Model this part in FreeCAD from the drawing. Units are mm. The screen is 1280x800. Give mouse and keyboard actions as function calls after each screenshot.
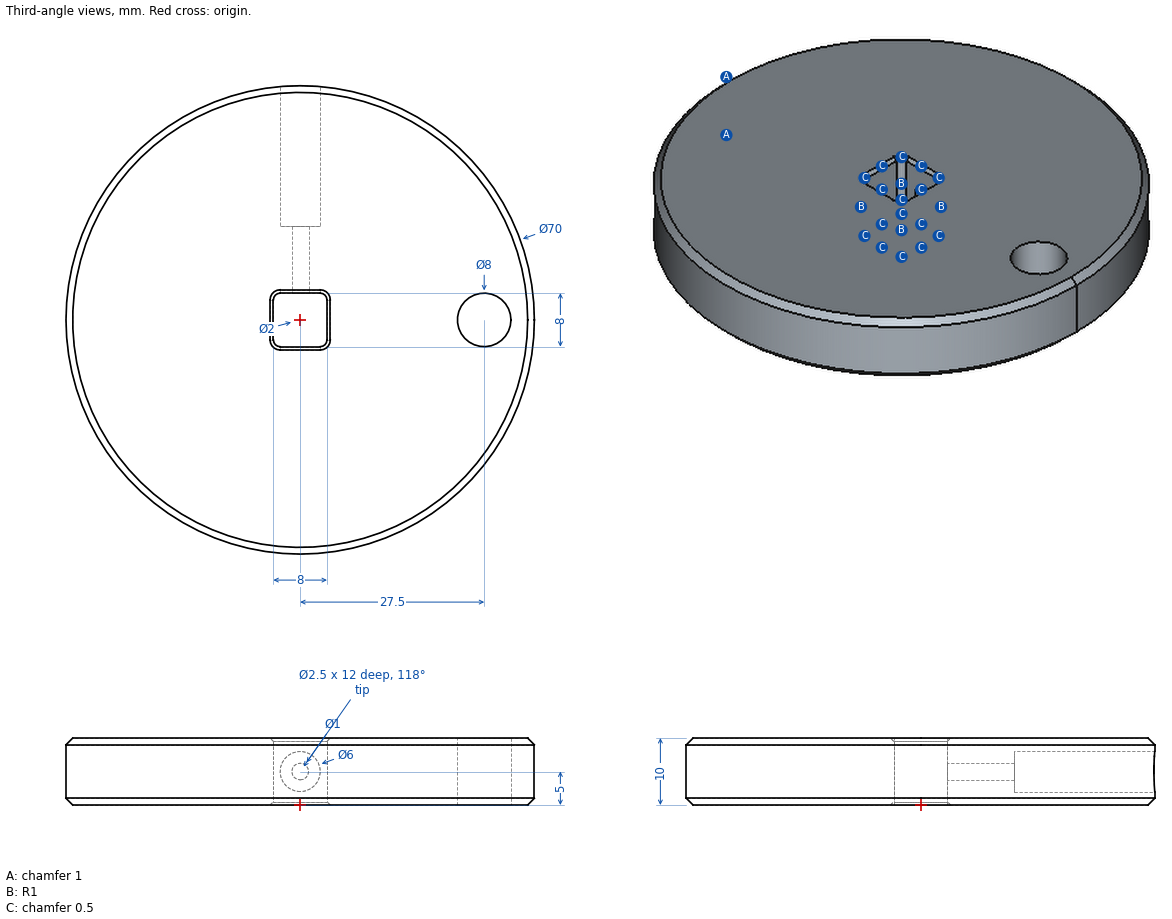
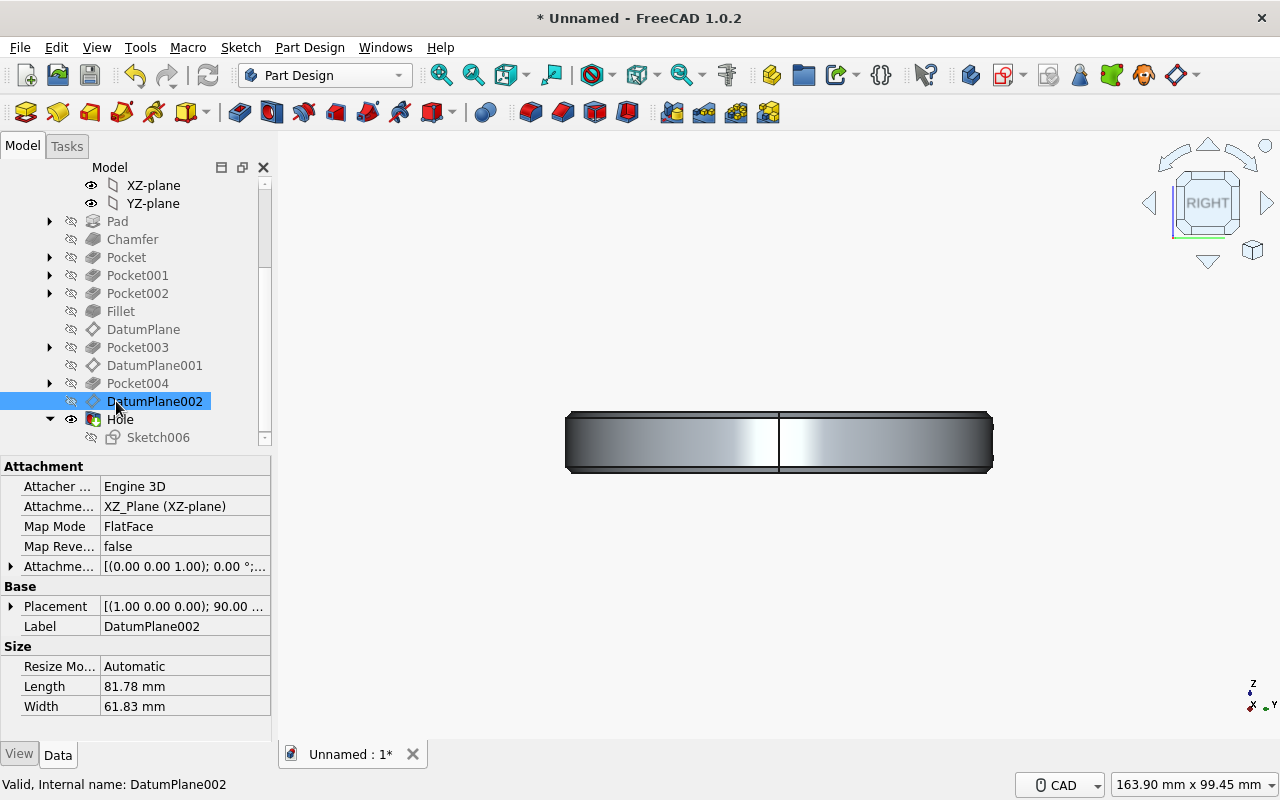
click(442, 76)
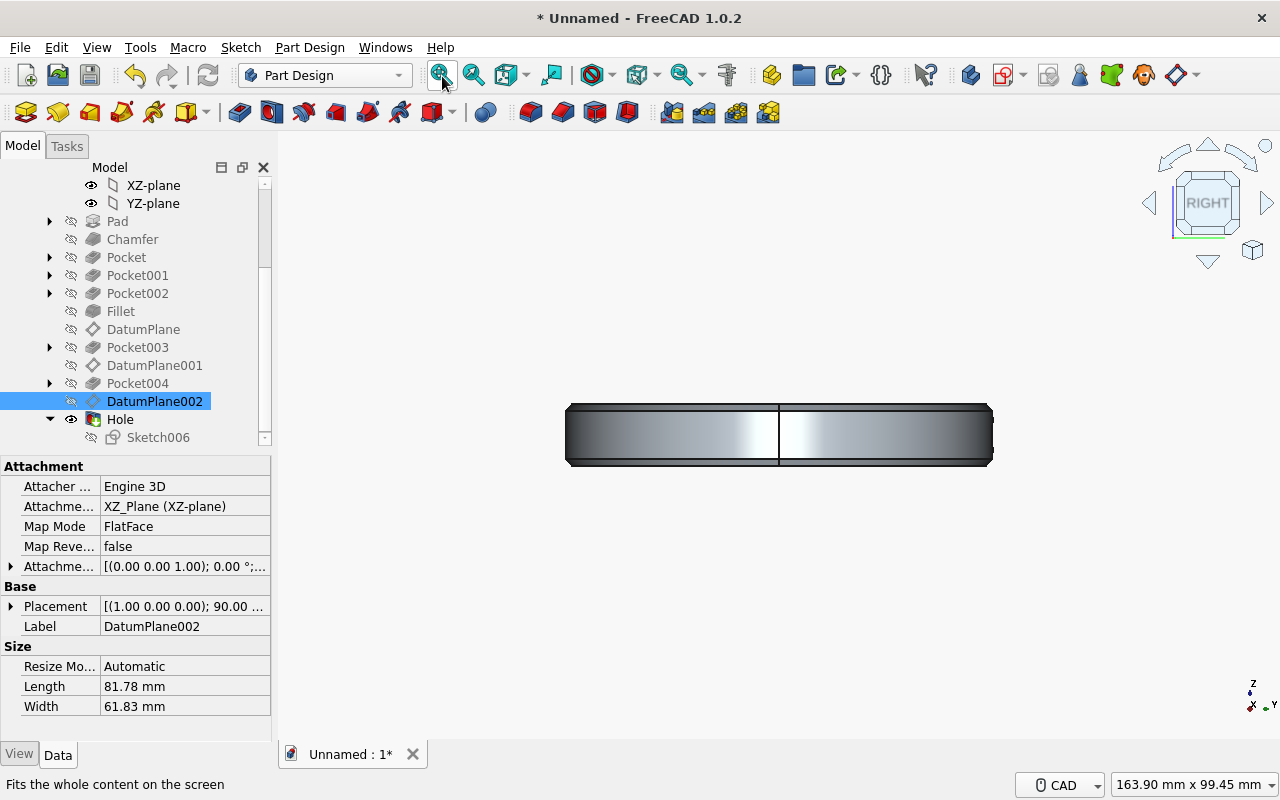
key(0)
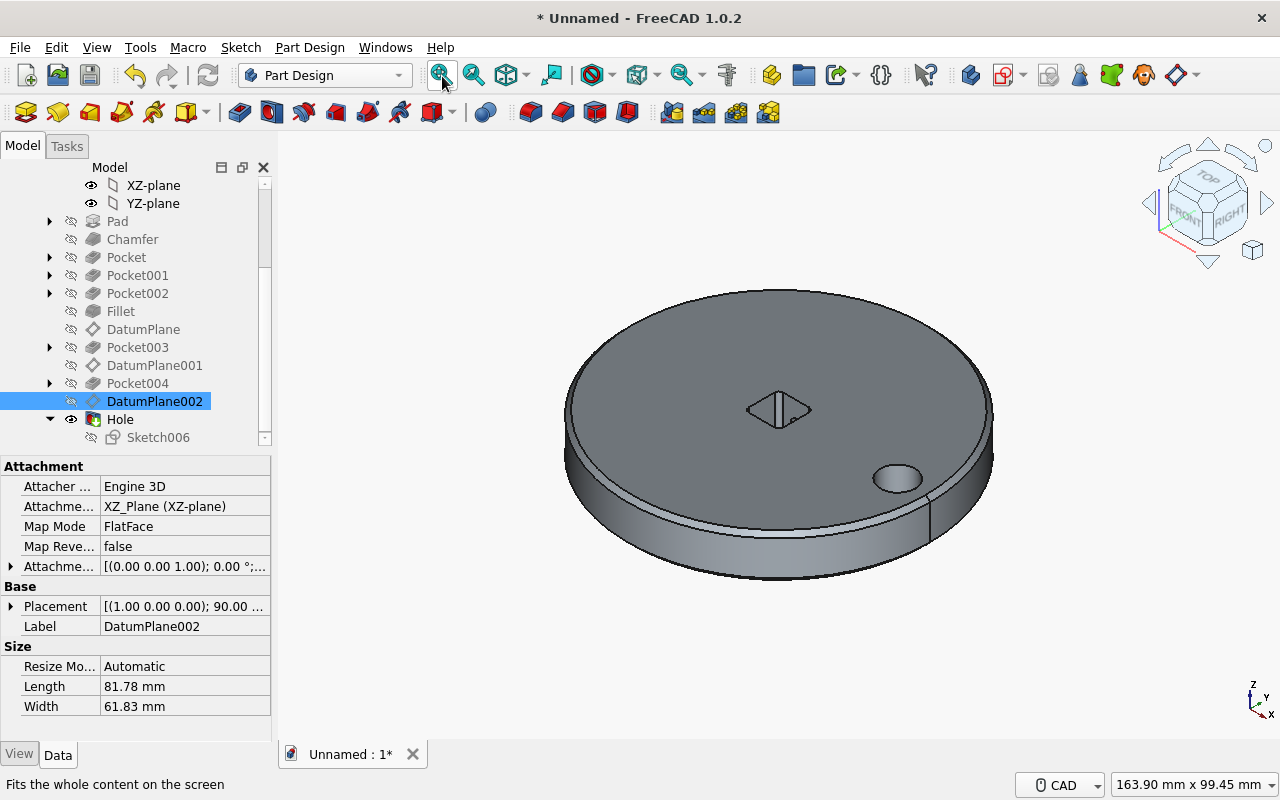
click(762, 399)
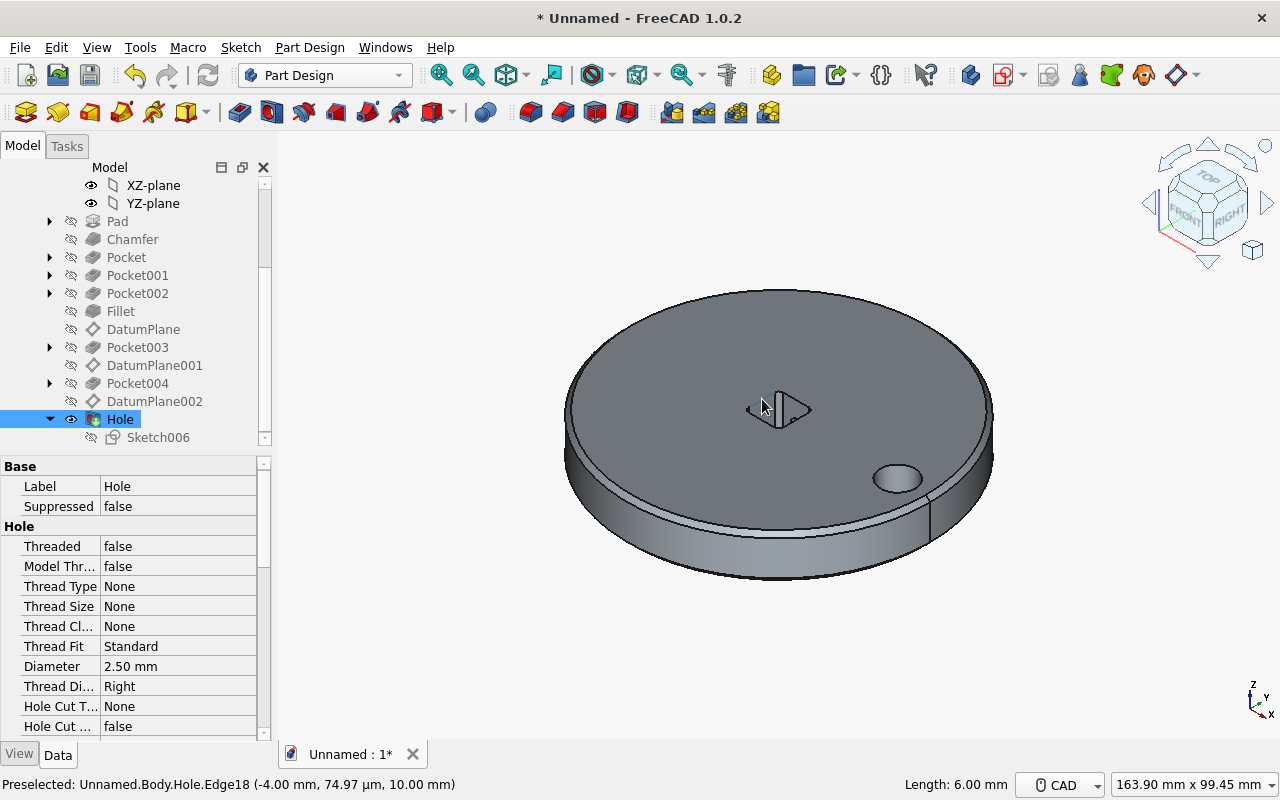
click(796, 399, ctrl)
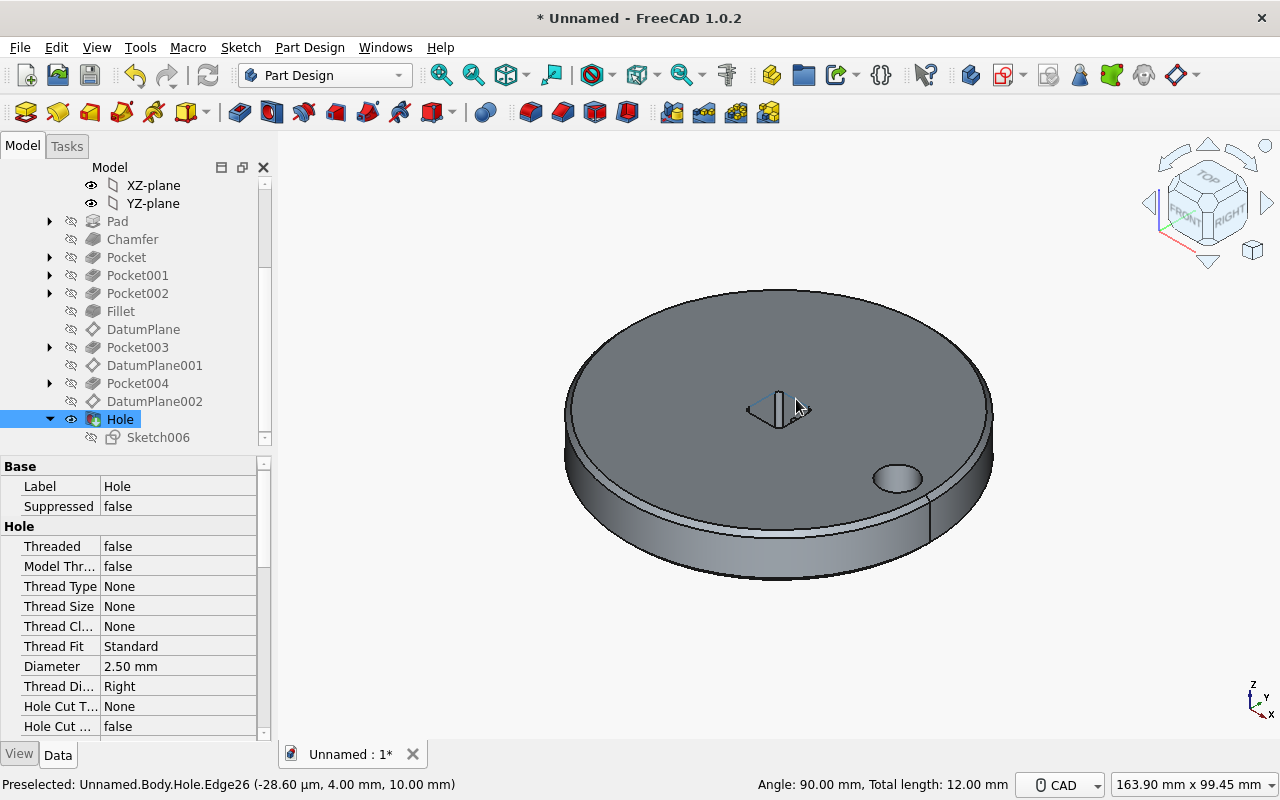
key(2)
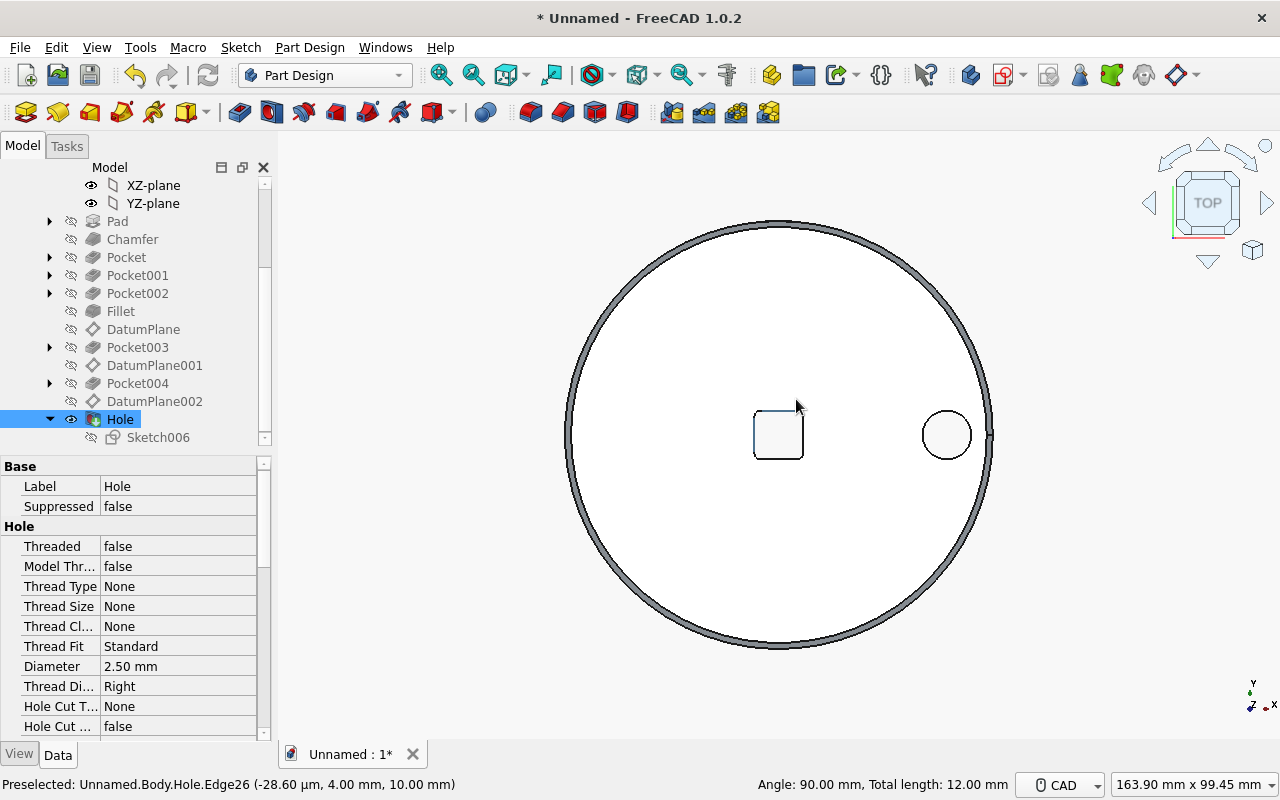
click(779, 458, ctrl)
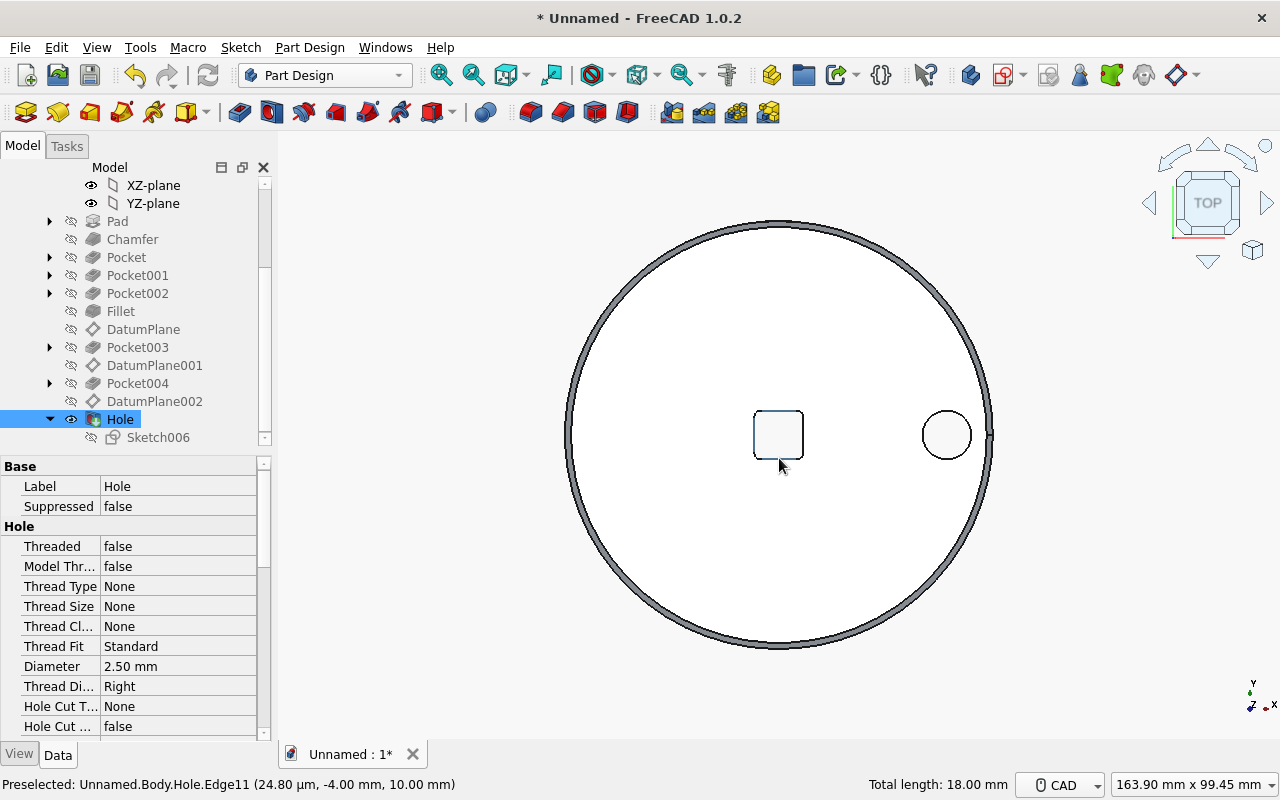
click(803, 434, ctrl)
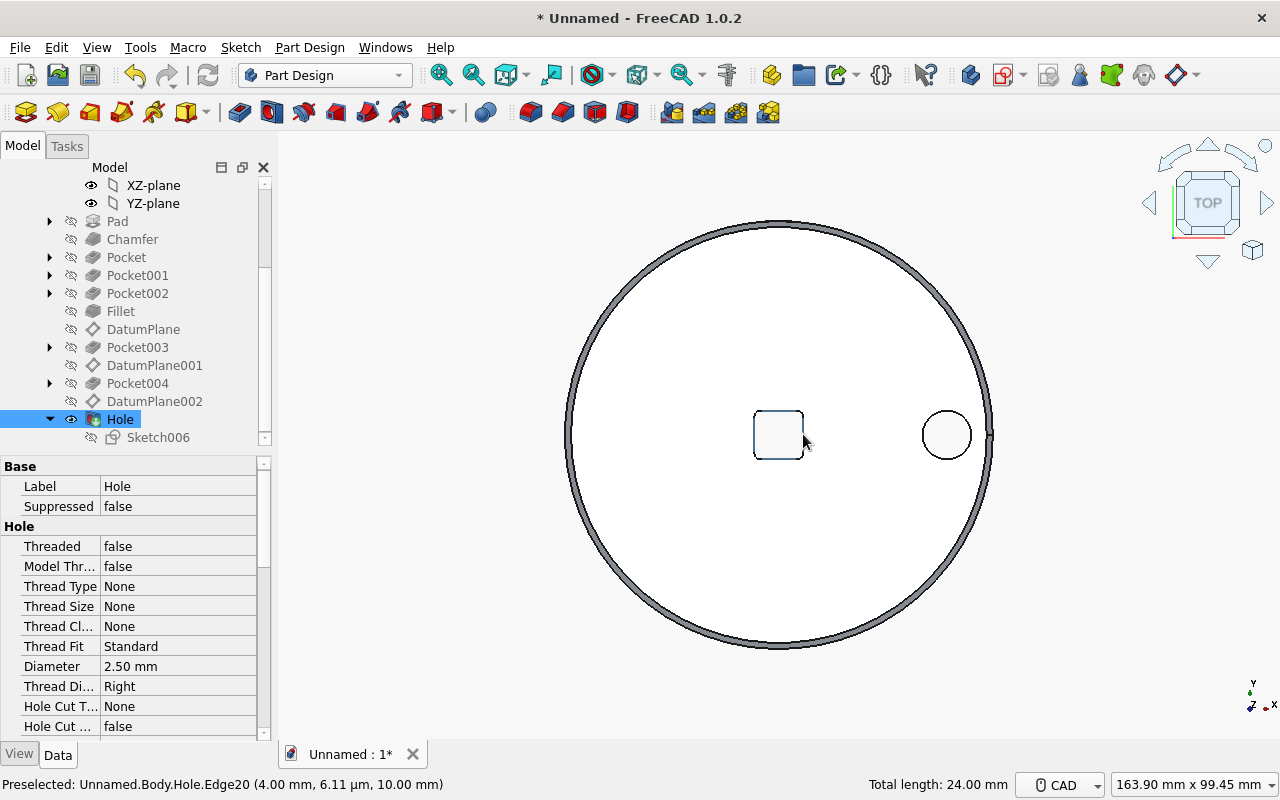
key(1)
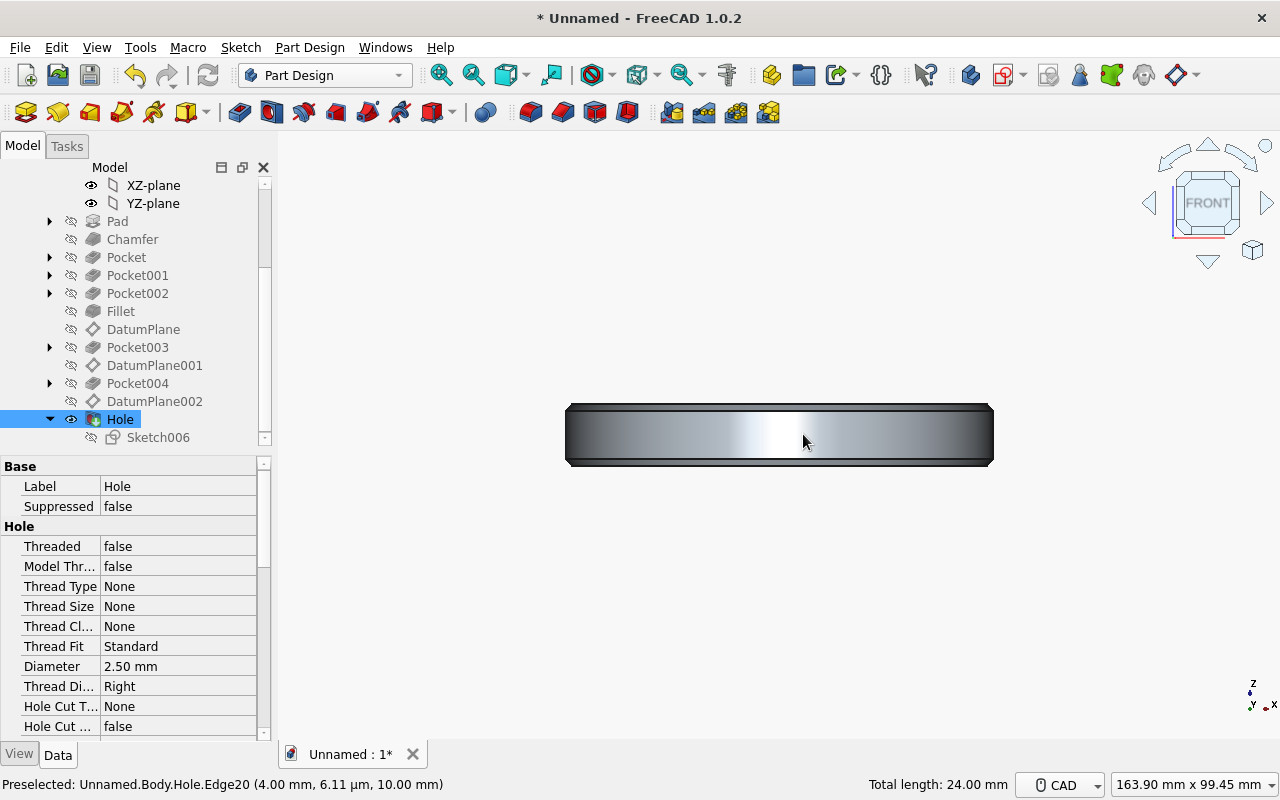
click(442, 76)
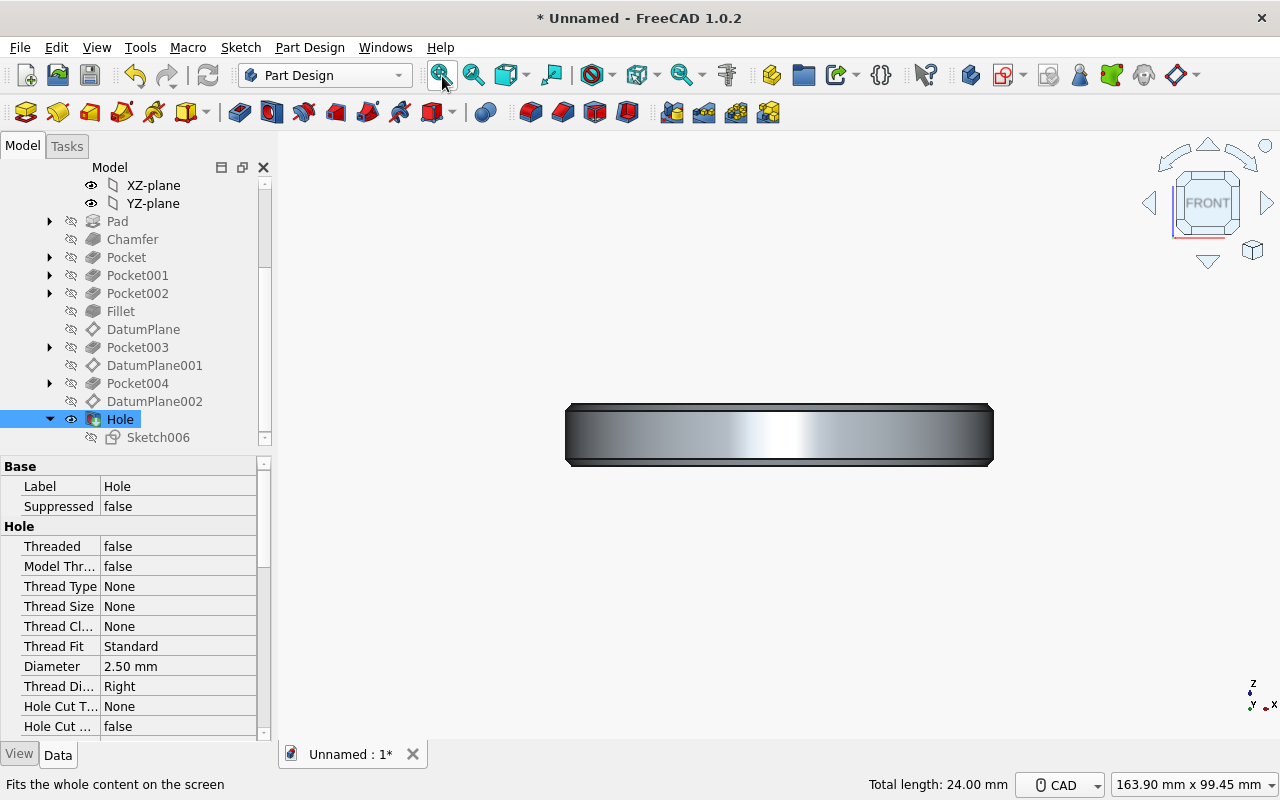
key(3)